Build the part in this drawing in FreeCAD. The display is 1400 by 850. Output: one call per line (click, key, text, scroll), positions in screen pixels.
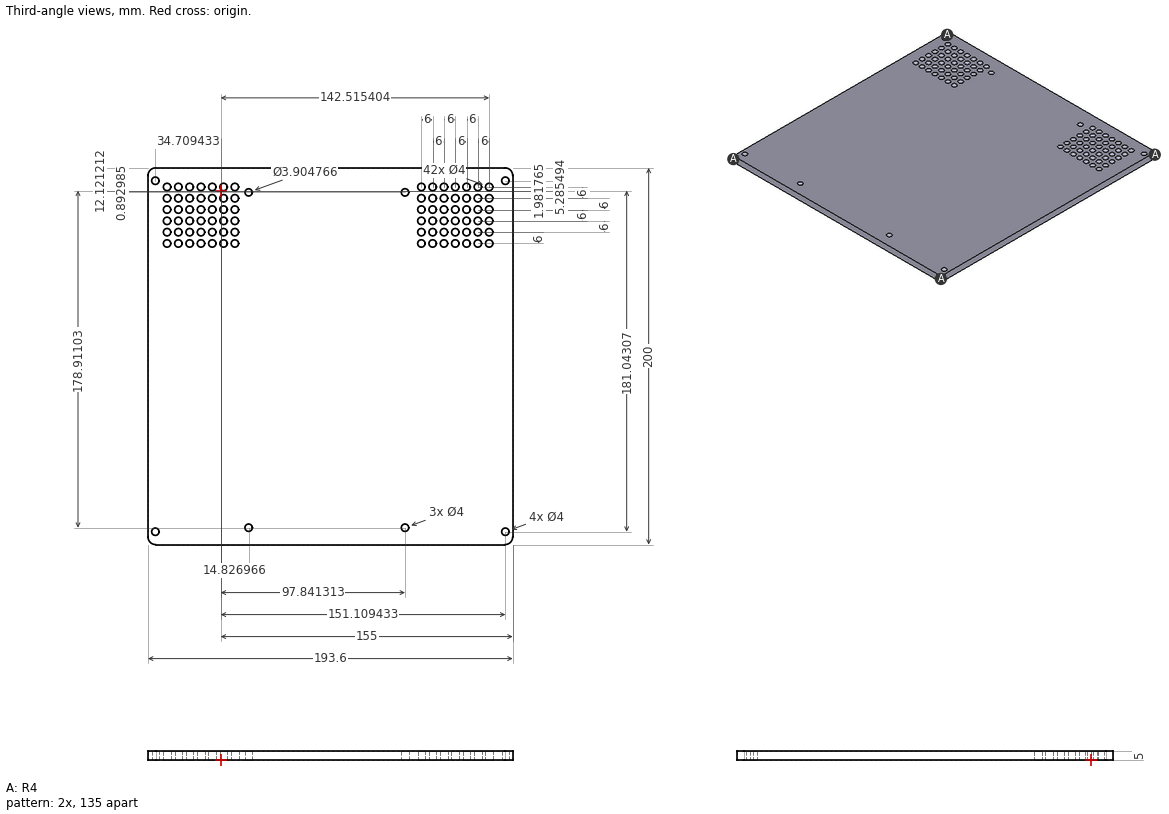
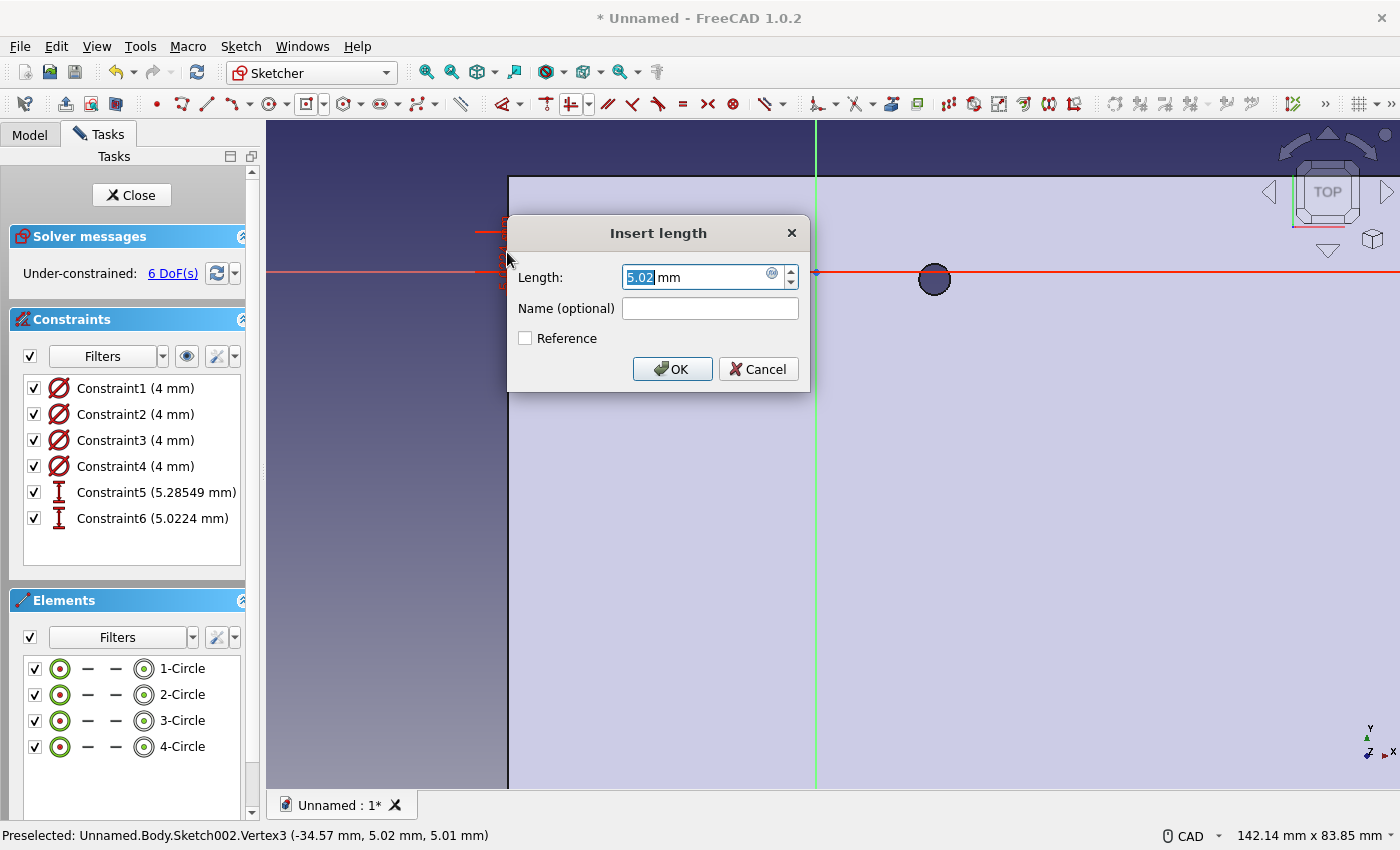
text(5.285494)
key(Return)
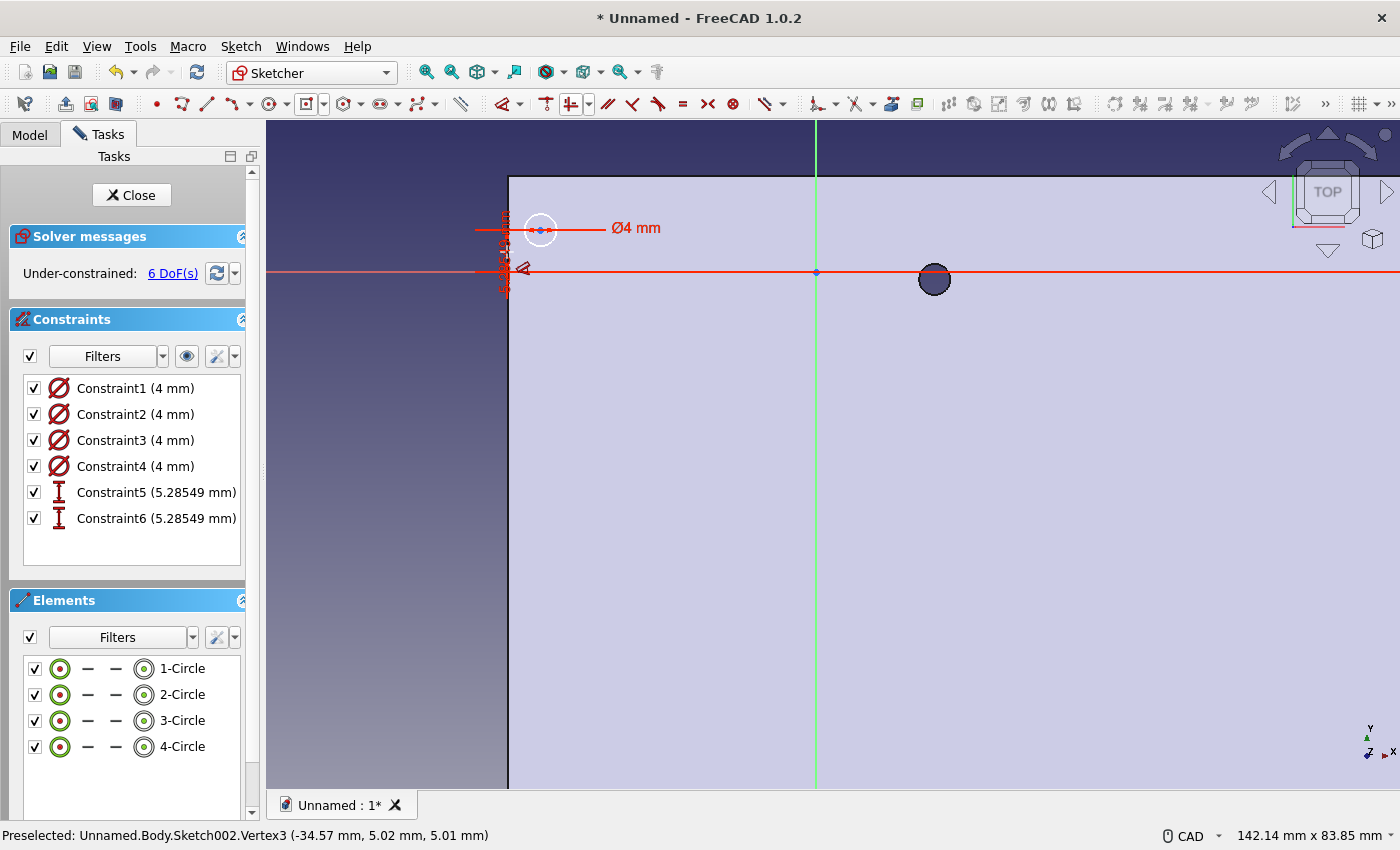
scroll(542, 231, down, 6)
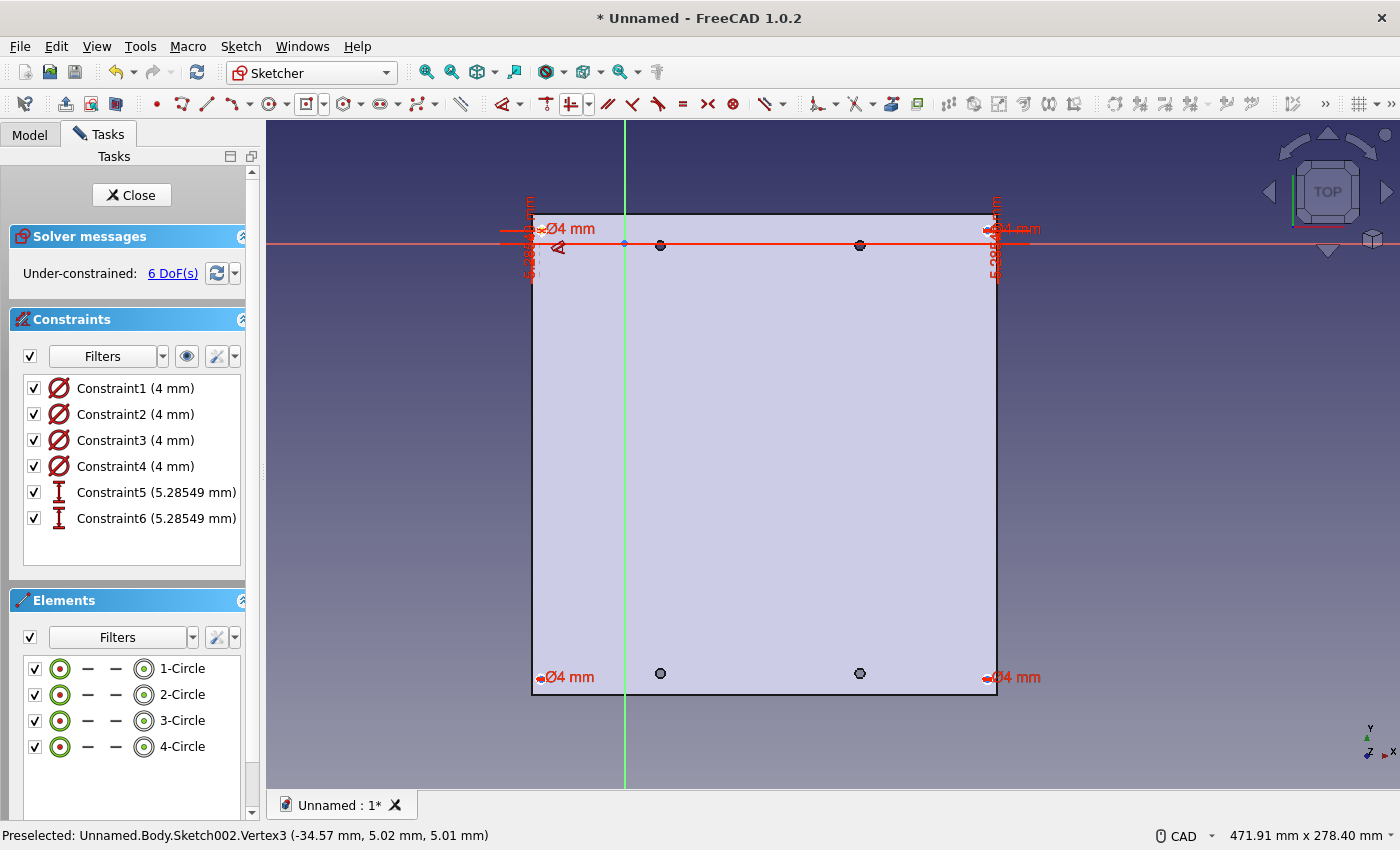
click(988, 679)
click(1022, 462)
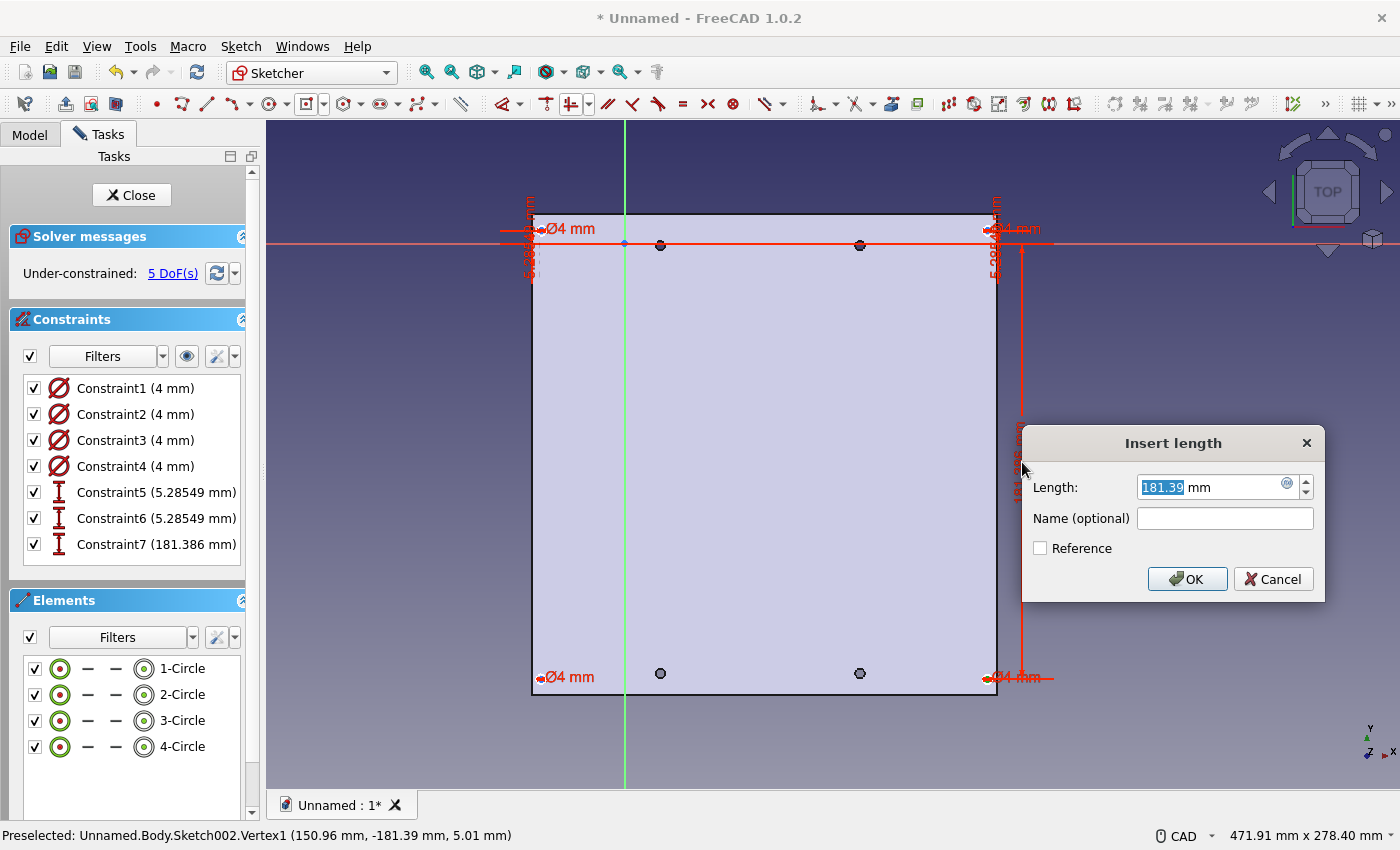
text(181.04307)
key(Return)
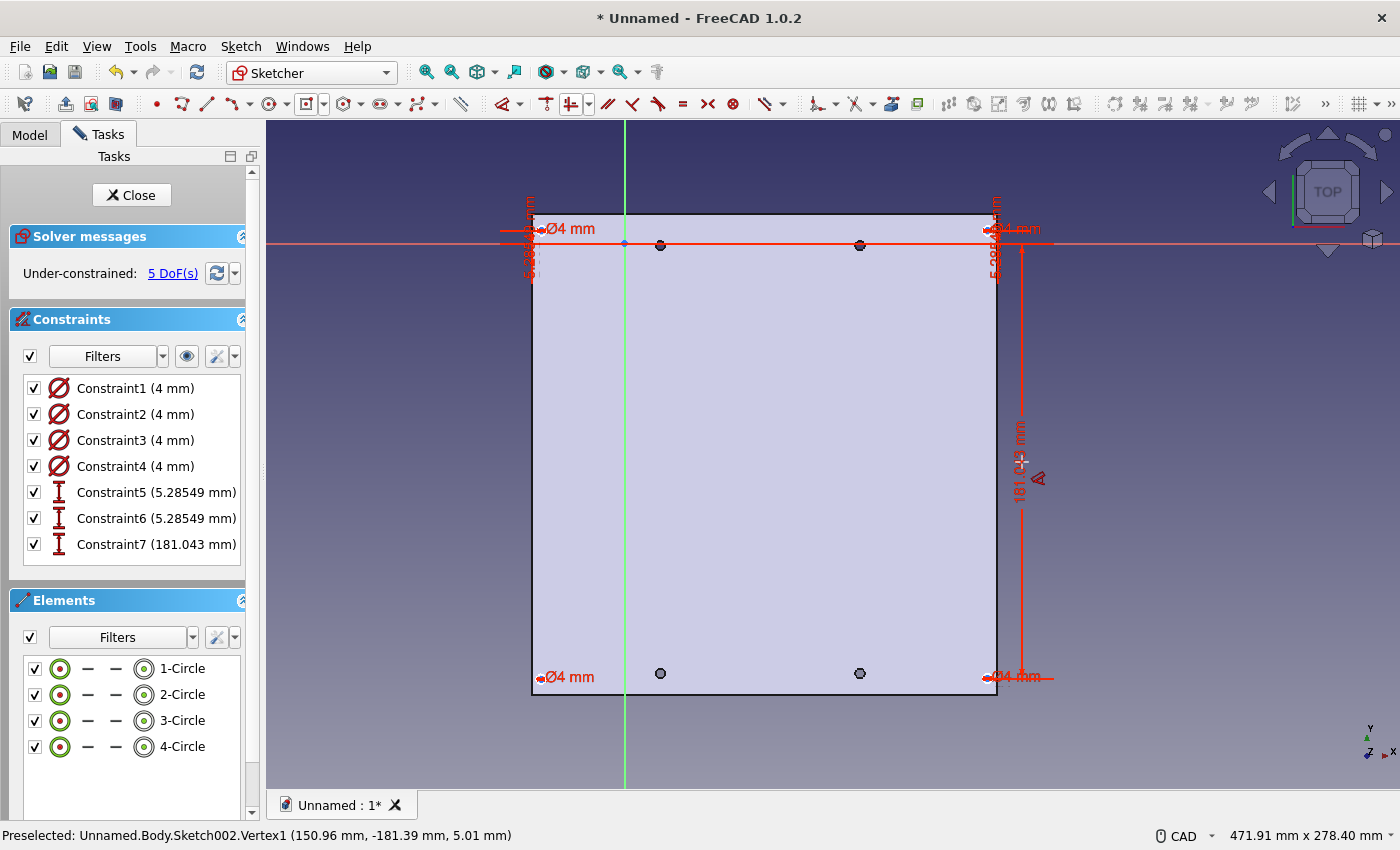
click(542, 231)
click(583, 197)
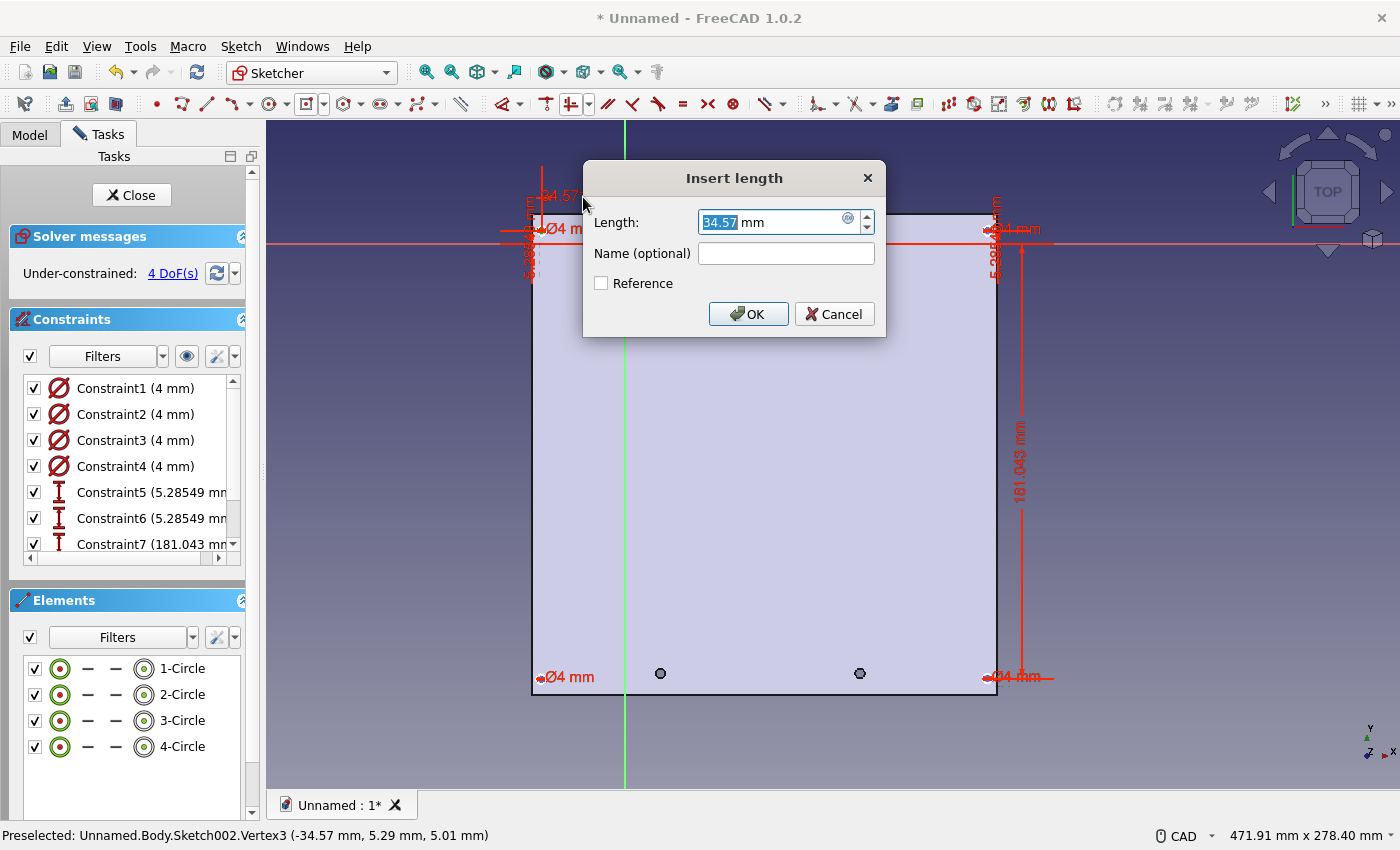
text(34.709433)
key(Return)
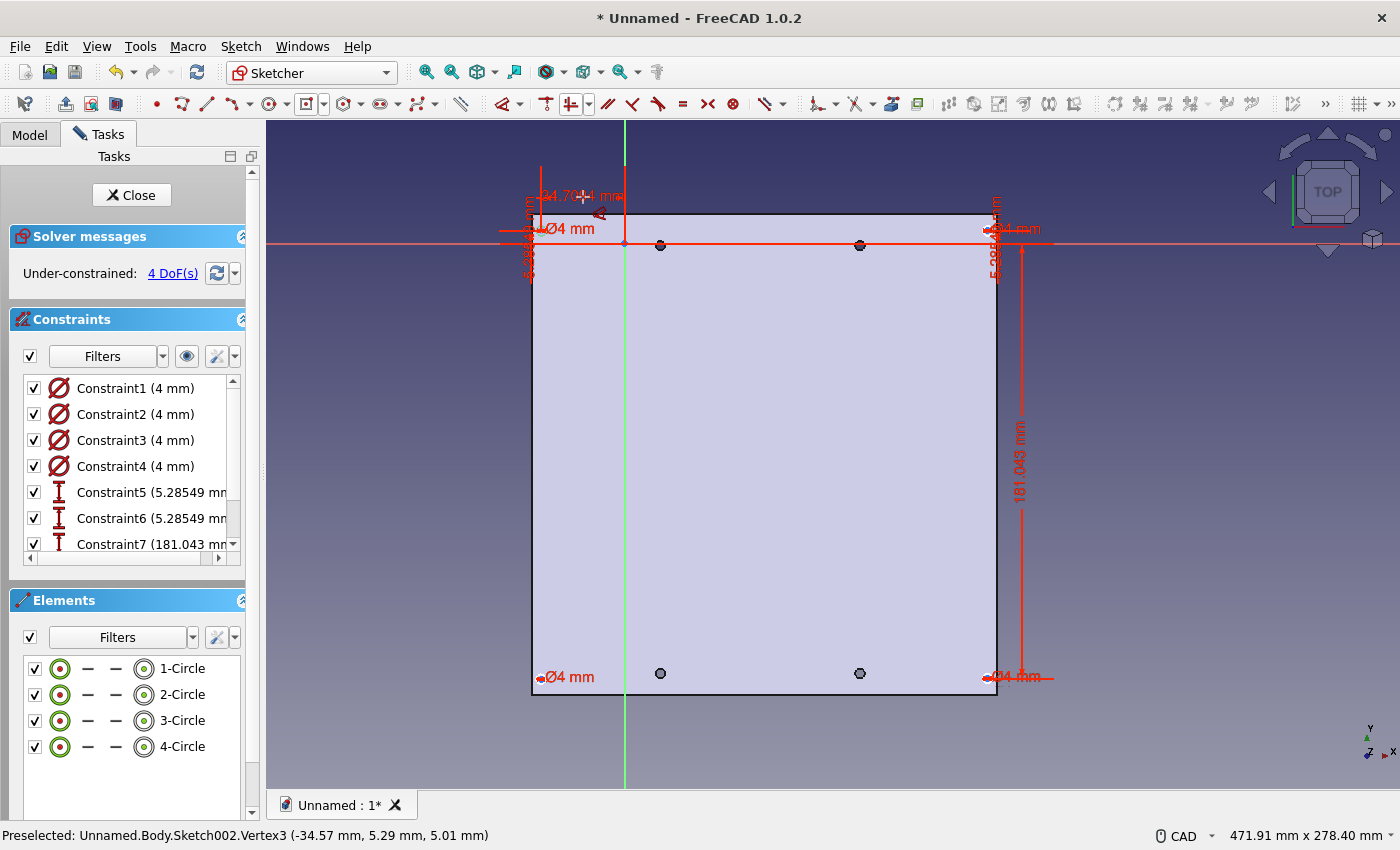
click(541, 679)
click(583, 713)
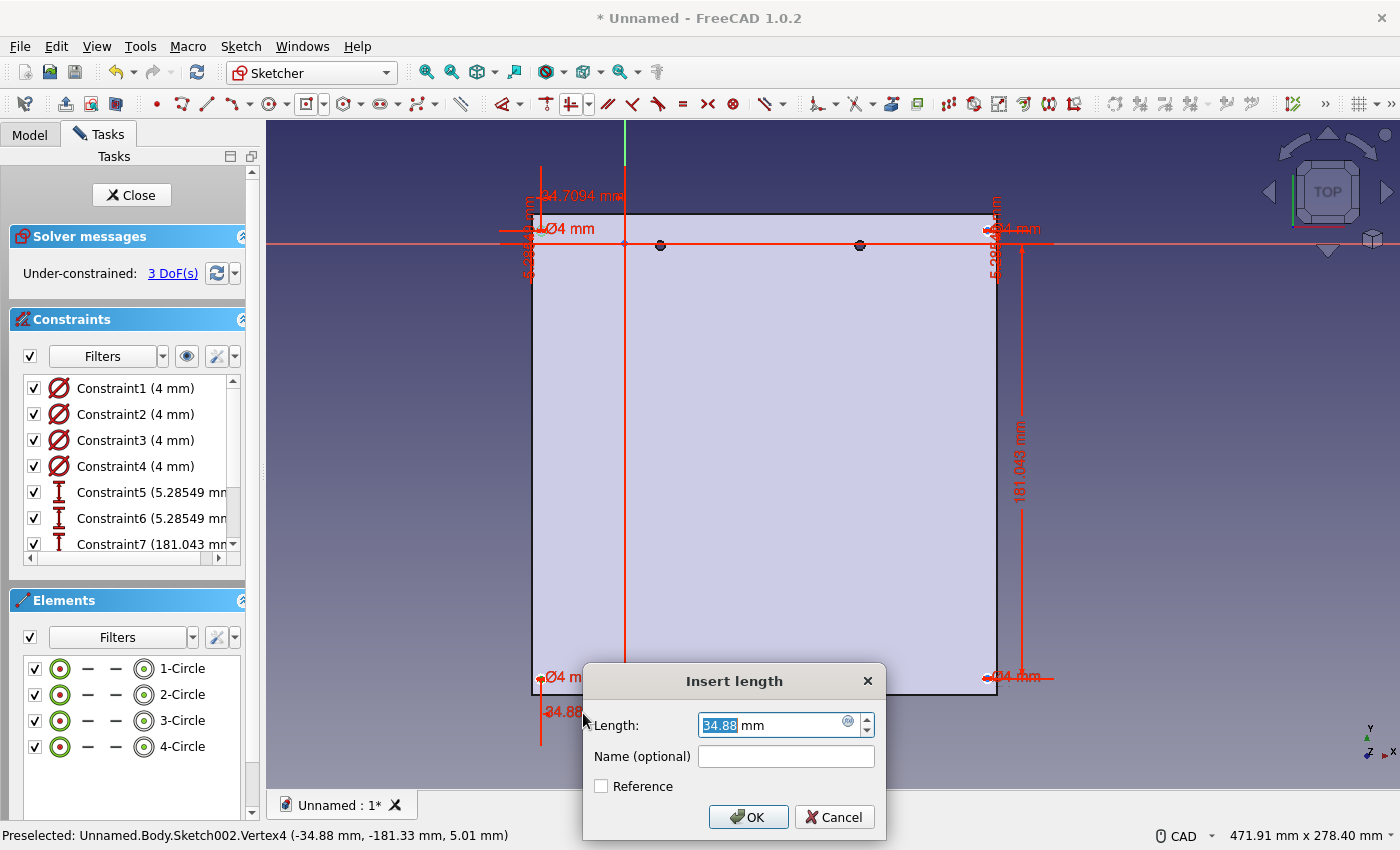
text(34.709433)
key(Return)